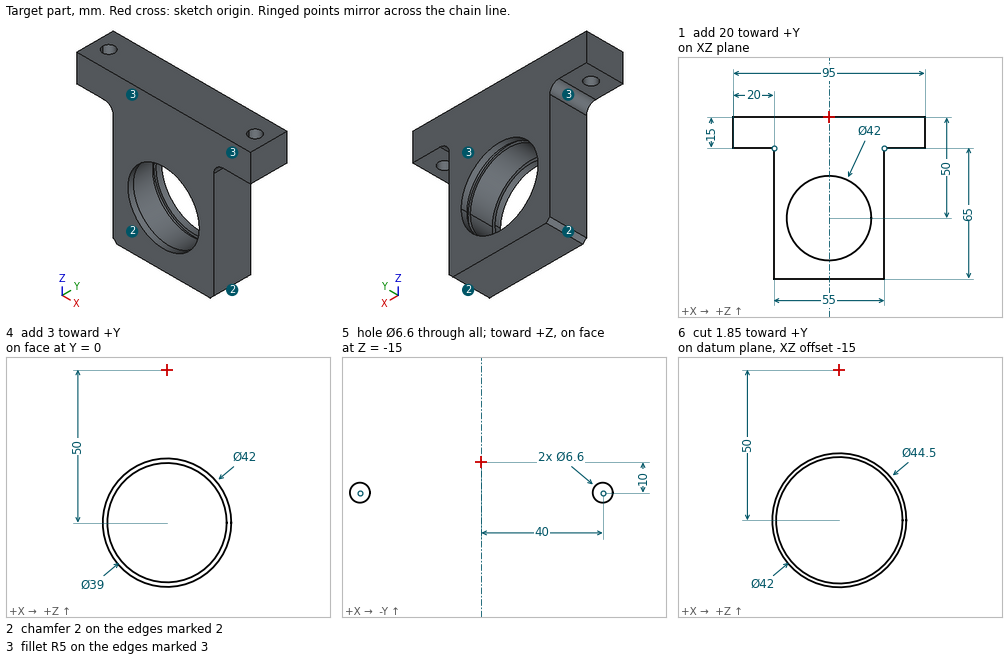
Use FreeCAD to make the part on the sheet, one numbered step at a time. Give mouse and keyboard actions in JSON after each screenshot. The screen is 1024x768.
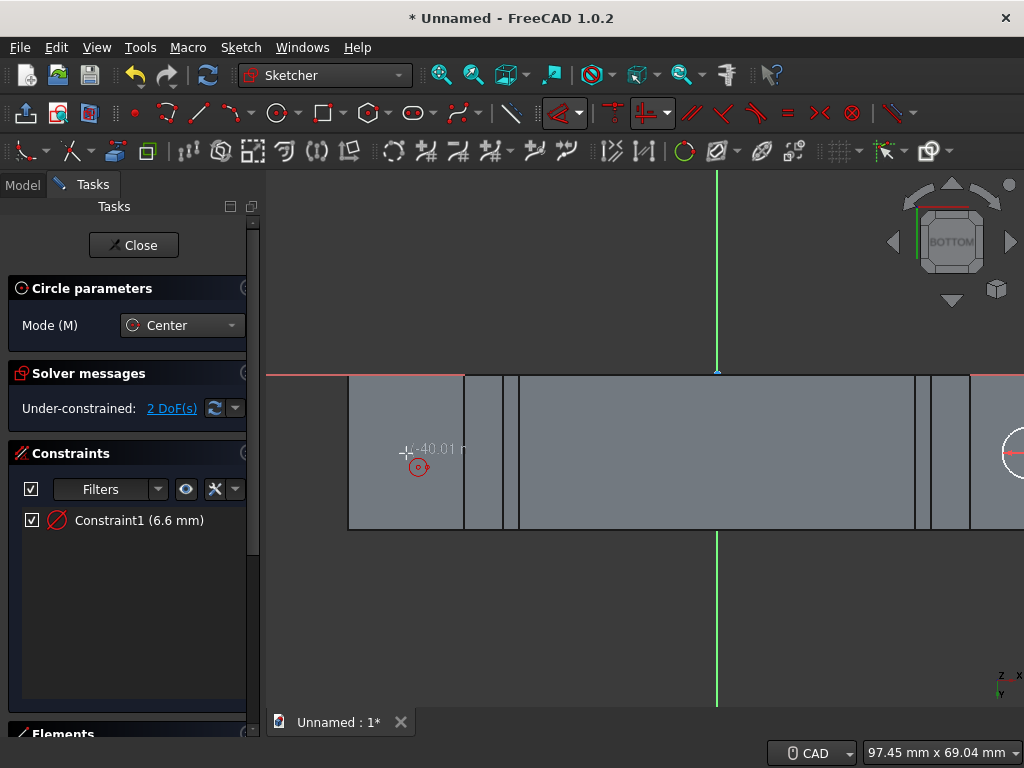
{"action": "left_click", "coordinate": [406, 453]}
{"action": "mouse_move", "coordinate": [424, 434]}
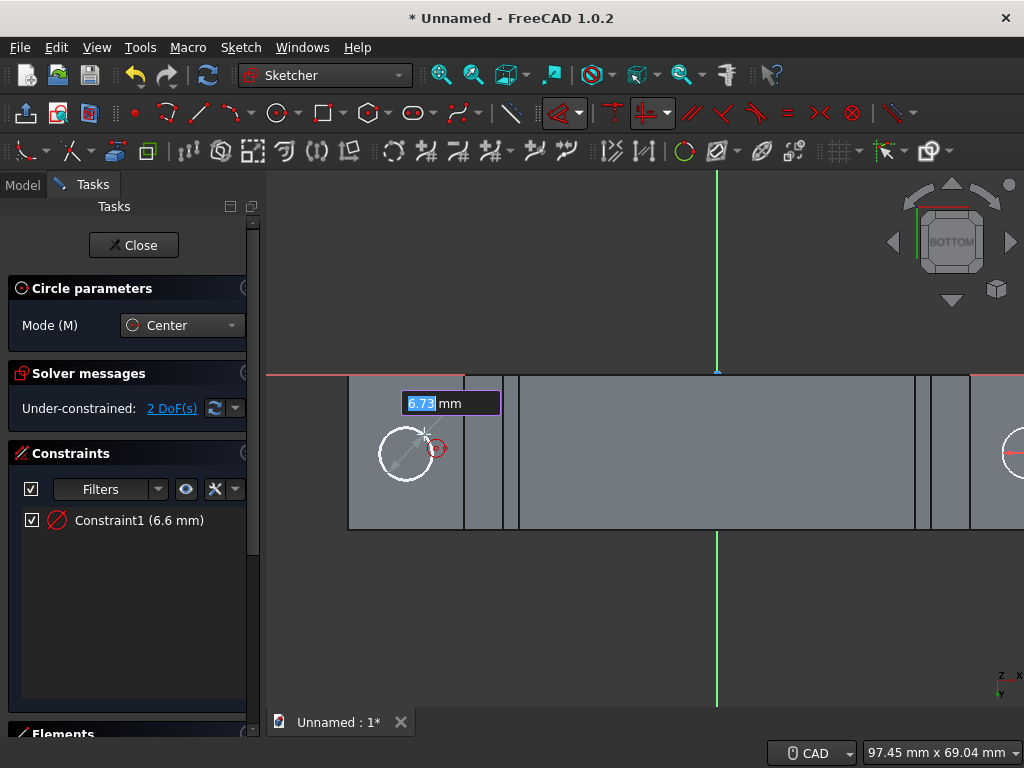
{"action": "type", "text": "6.6"}
{"action": "key", "text": "Return"}
{"action": "key", "text": "Escape"}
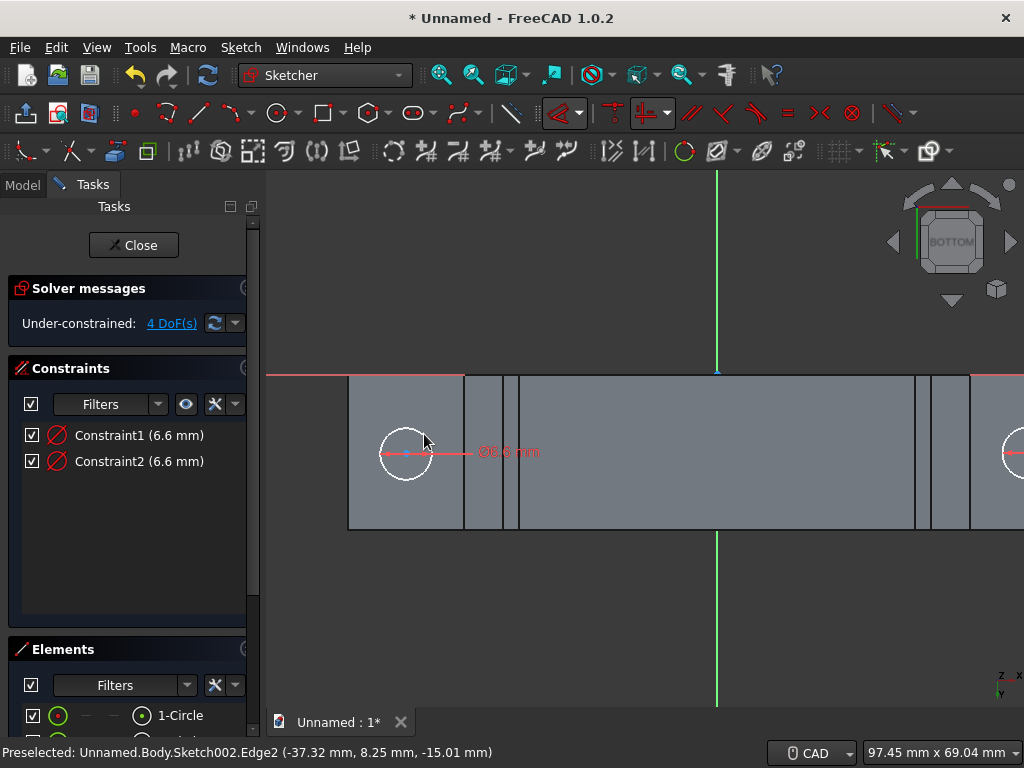
{"action": "scroll", "coordinate": [406, 453], "scroll_direction": "down", "scroll_amount": 3}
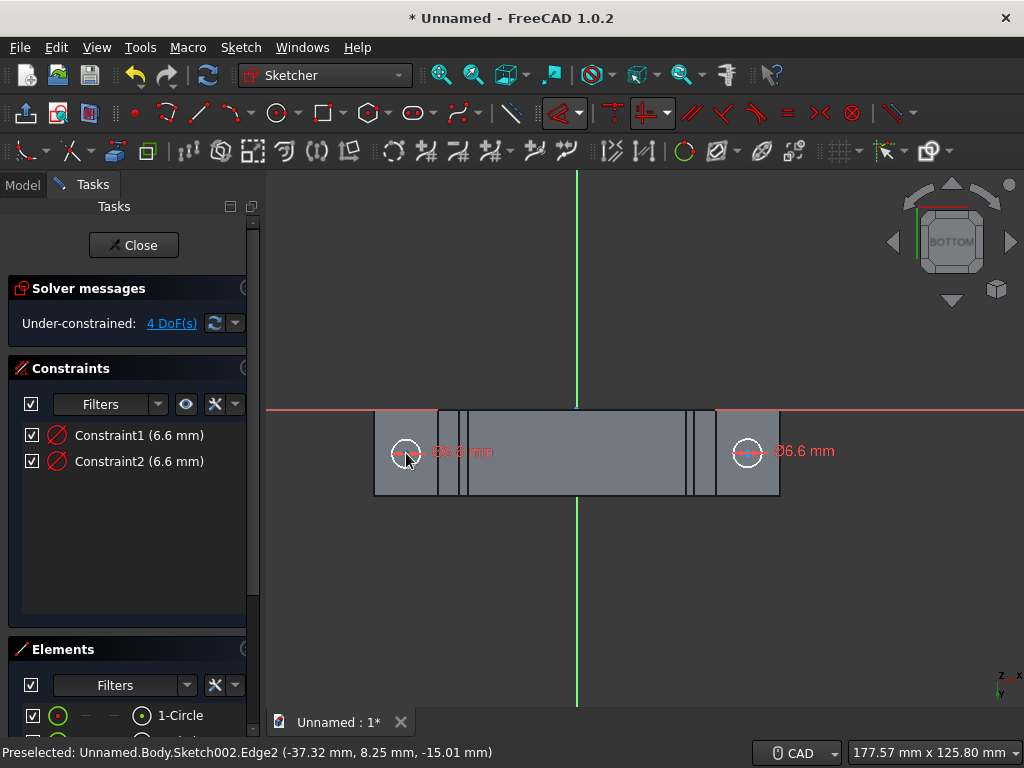
{"action": "left_click", "coordinate": [748, 453]}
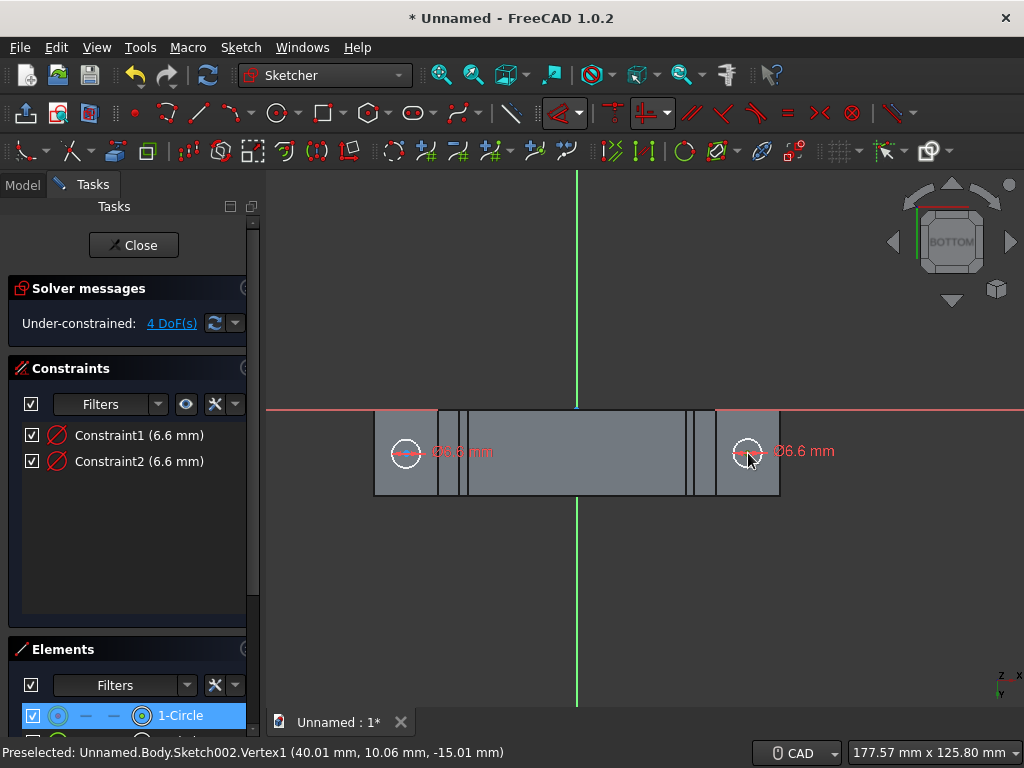
{"action": "left_click", "coordinate": [406, 454]}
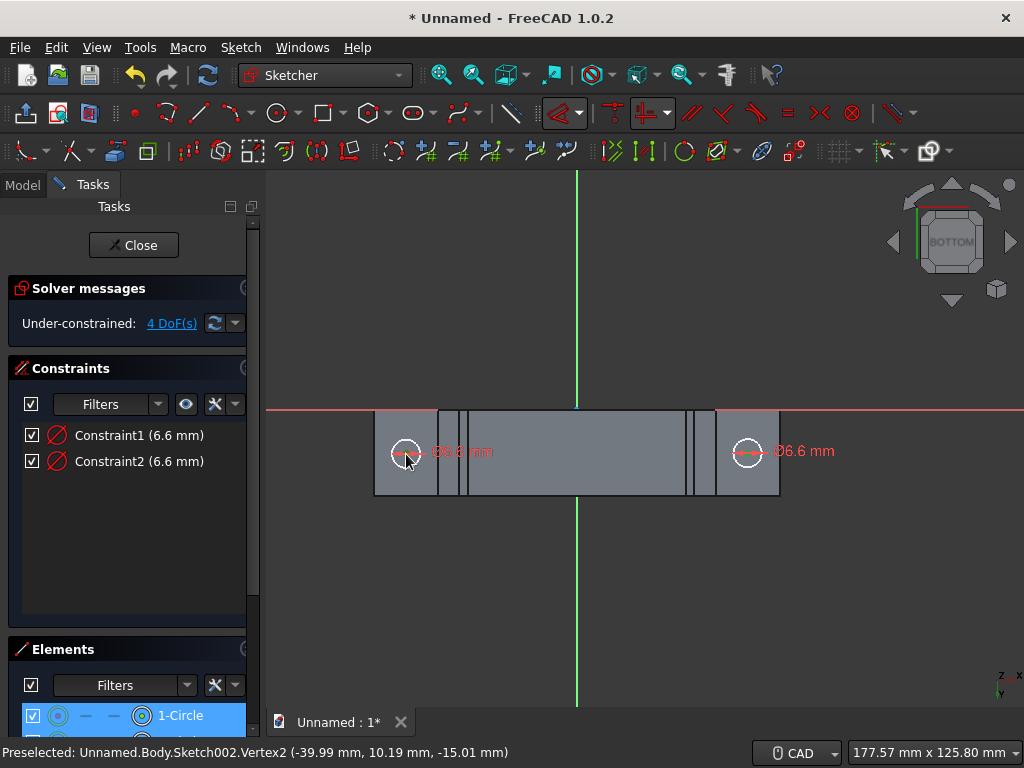
{"action": "left_click", "coordinate": [577, 645]}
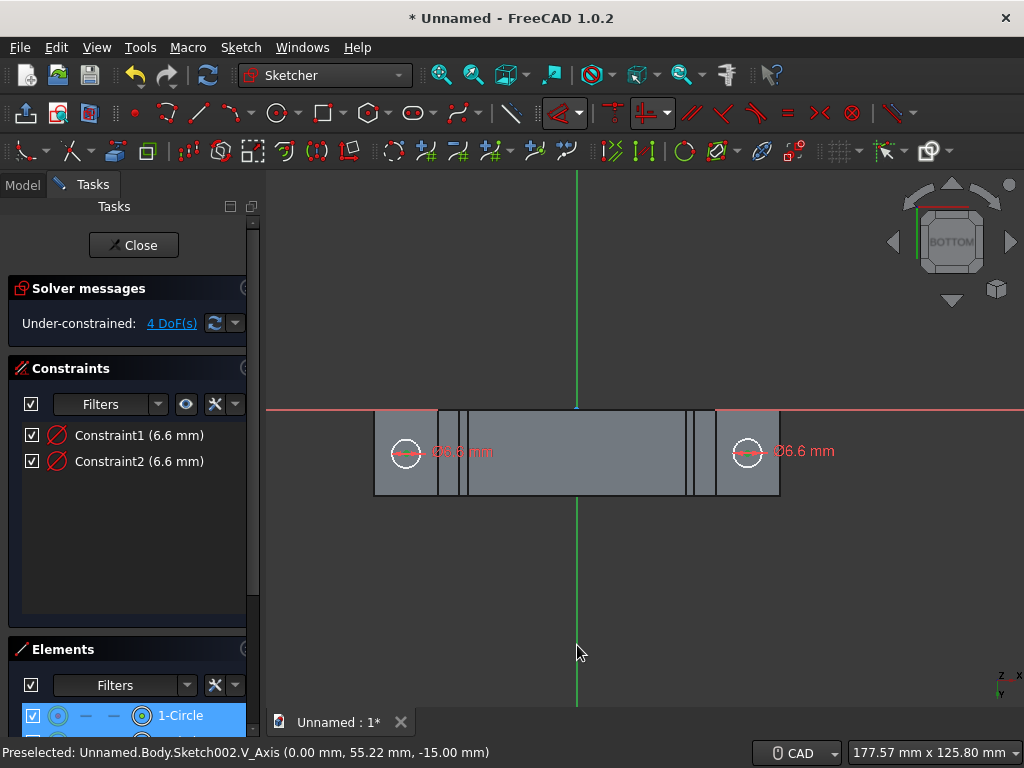
{"action": "left_click", "coordinate": [820, 114]}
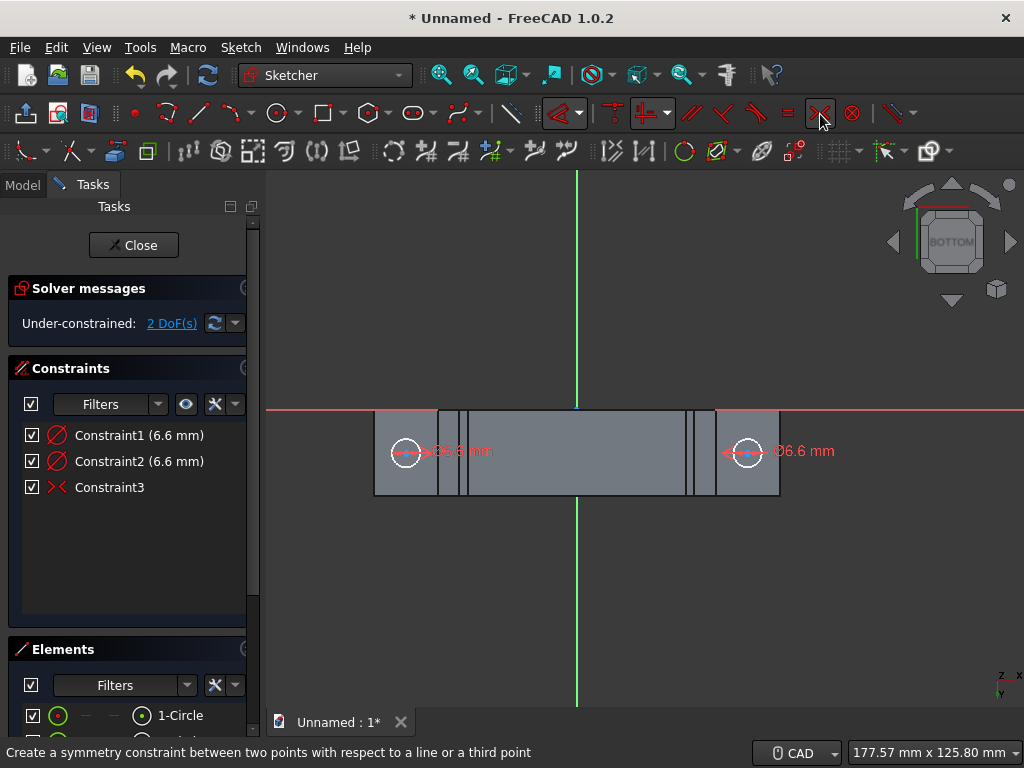
{"action": "left_click", "coordinate": [748, 453]}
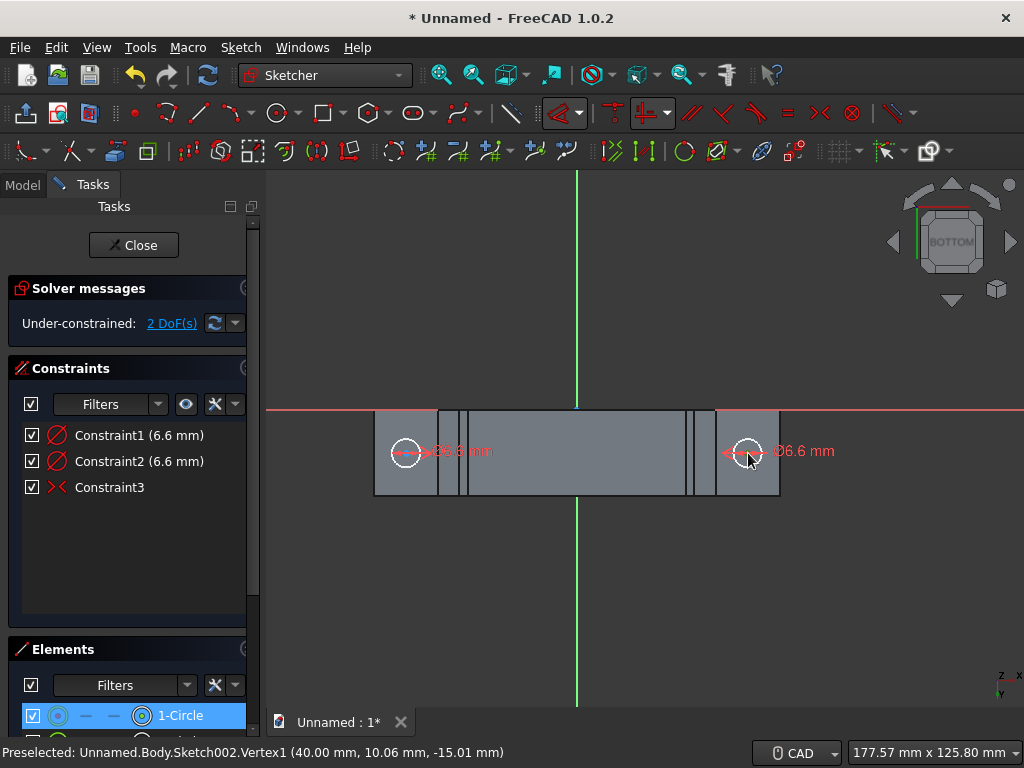
{"action": "key", "text": "l"}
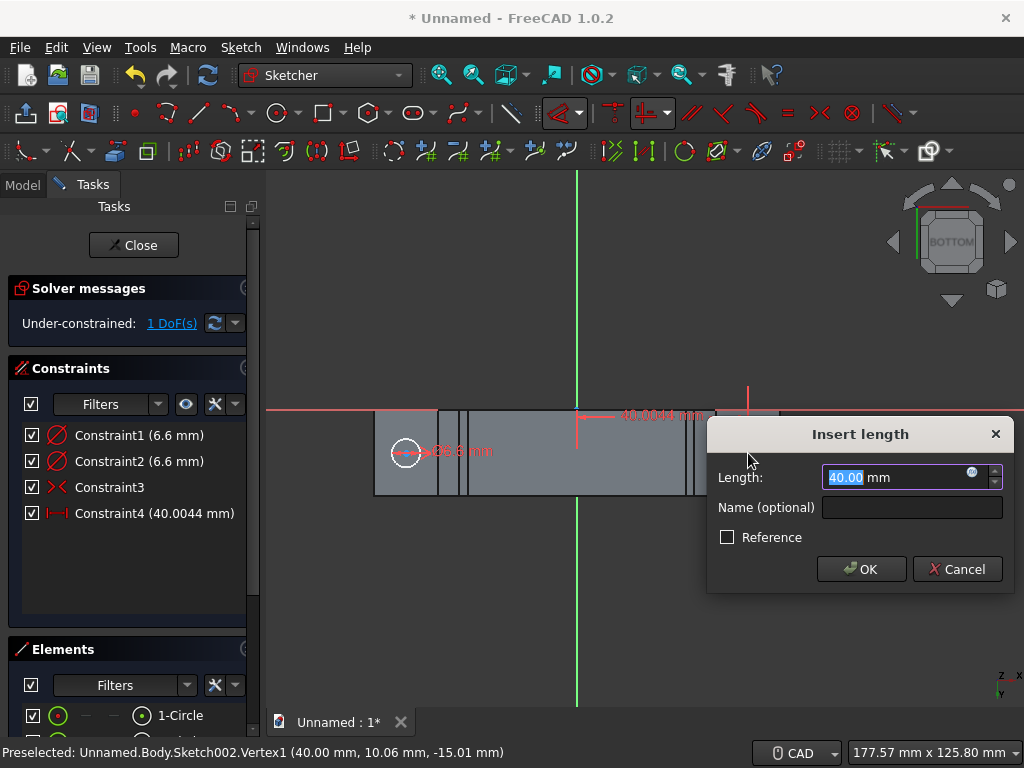
{"action": "type", "text": "40"}
{"action": "key", "text": "Return"}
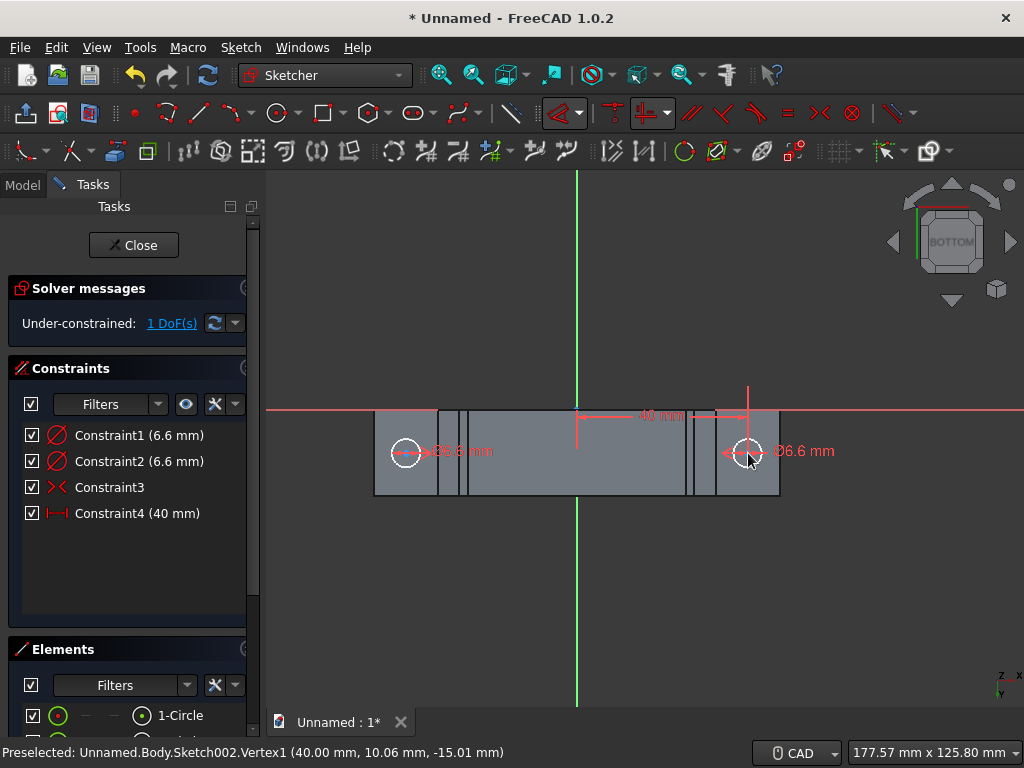
{"action": "left_click", "coordinate": [748, 453]}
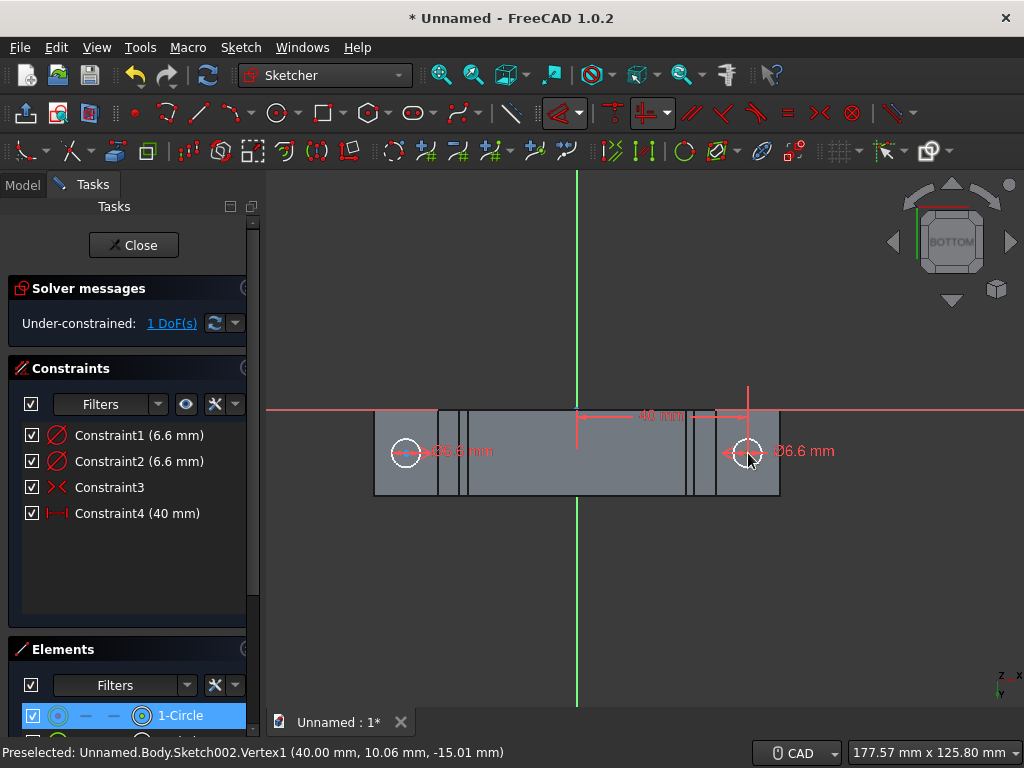
{"action": "key", "text": "i"}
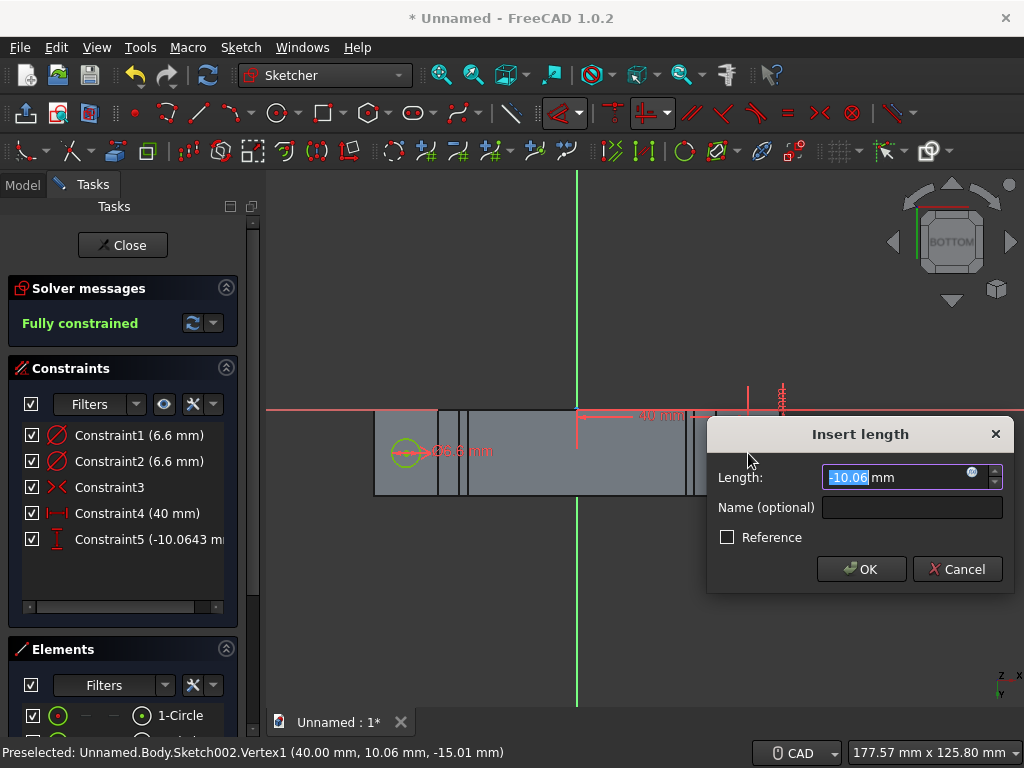
{"action": "type", "text": "-10"}
{"action": "key", "text": "Return"}